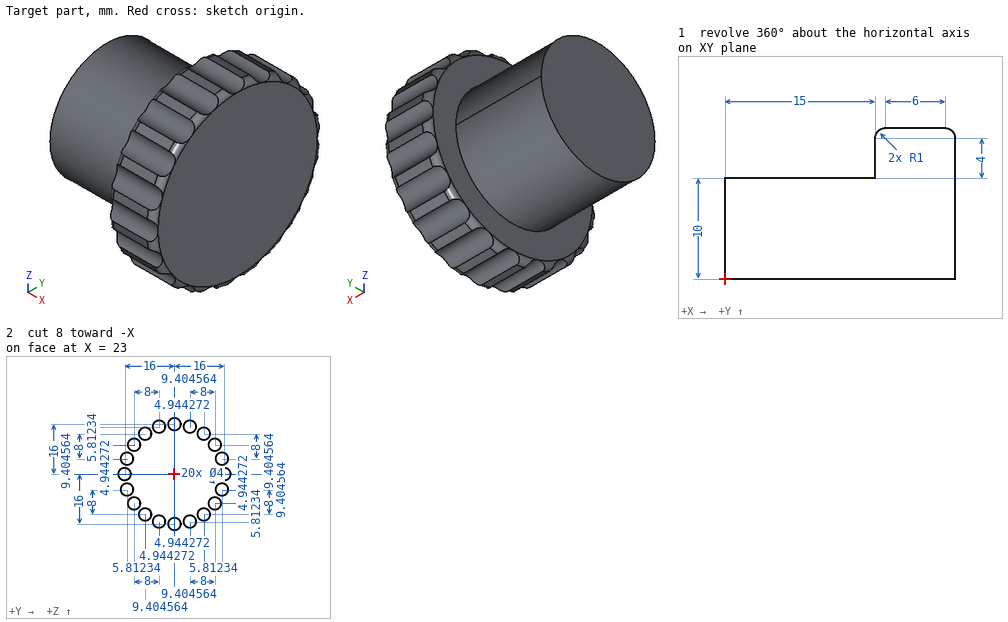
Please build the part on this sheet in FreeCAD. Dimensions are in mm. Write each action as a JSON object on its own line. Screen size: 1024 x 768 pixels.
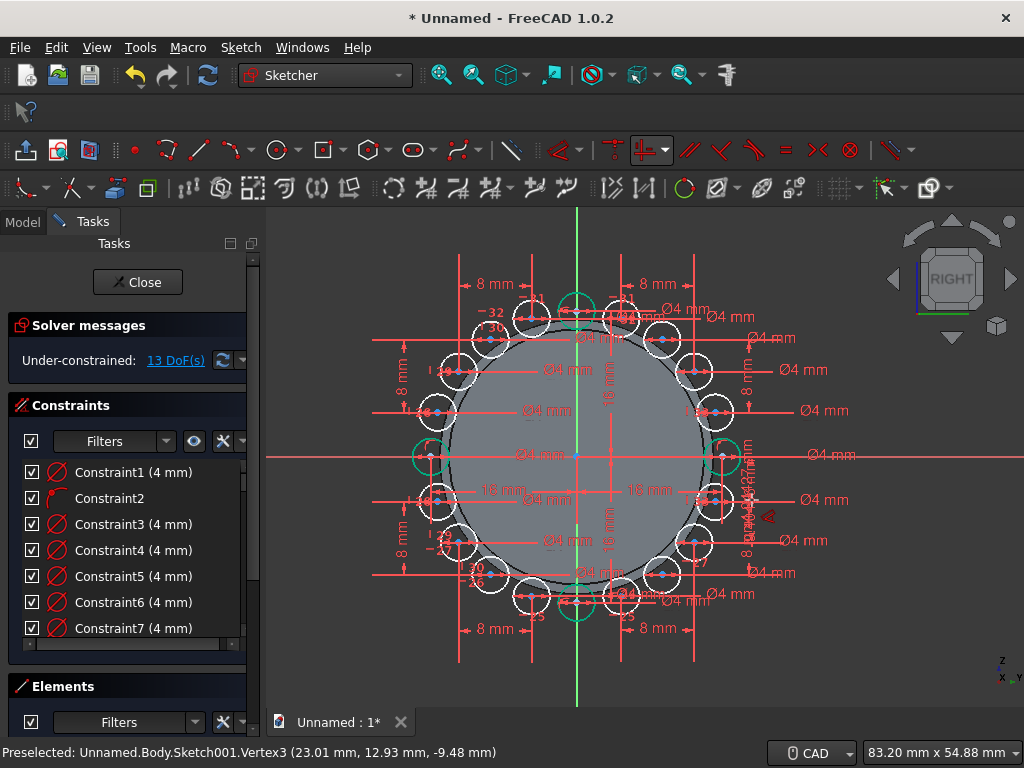
{"action": "left_click", "coordinate": [662, 575]}
{"action": "left_click", "coordinate": [619, 423]}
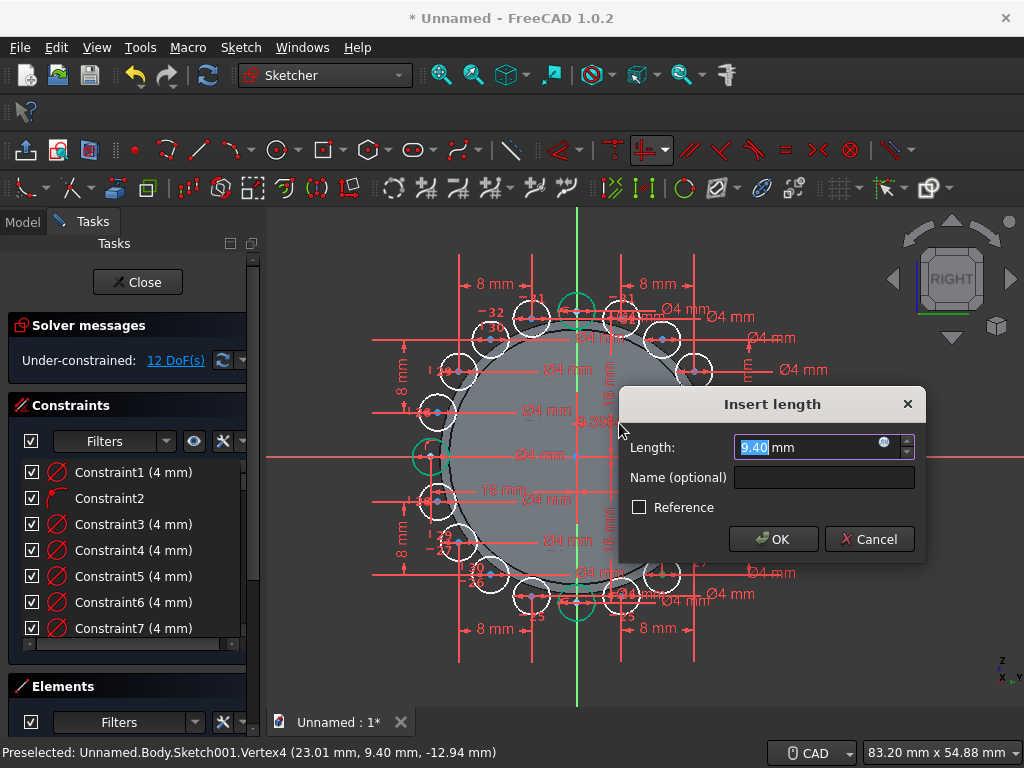
{"action": "type", "text": "9.404564"}
{"action": "key", "text": "Return"}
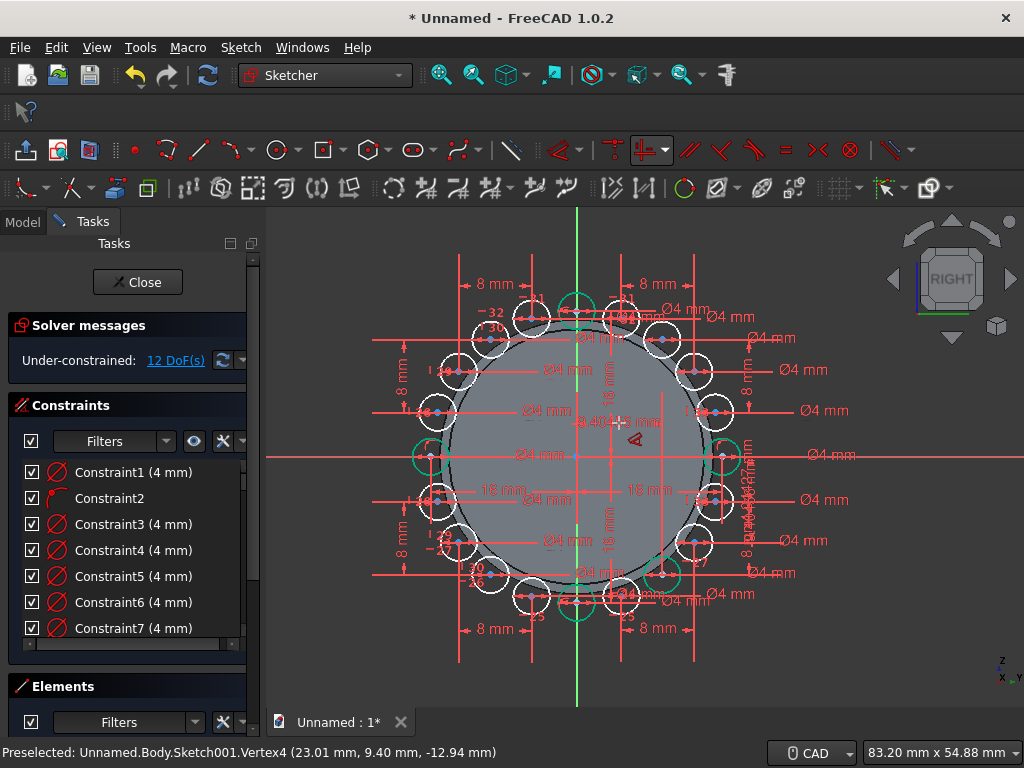
{"action": "left_click", "coordinate": [621, 596]}
{"action": "left_click", "coordinate": [599, 654]}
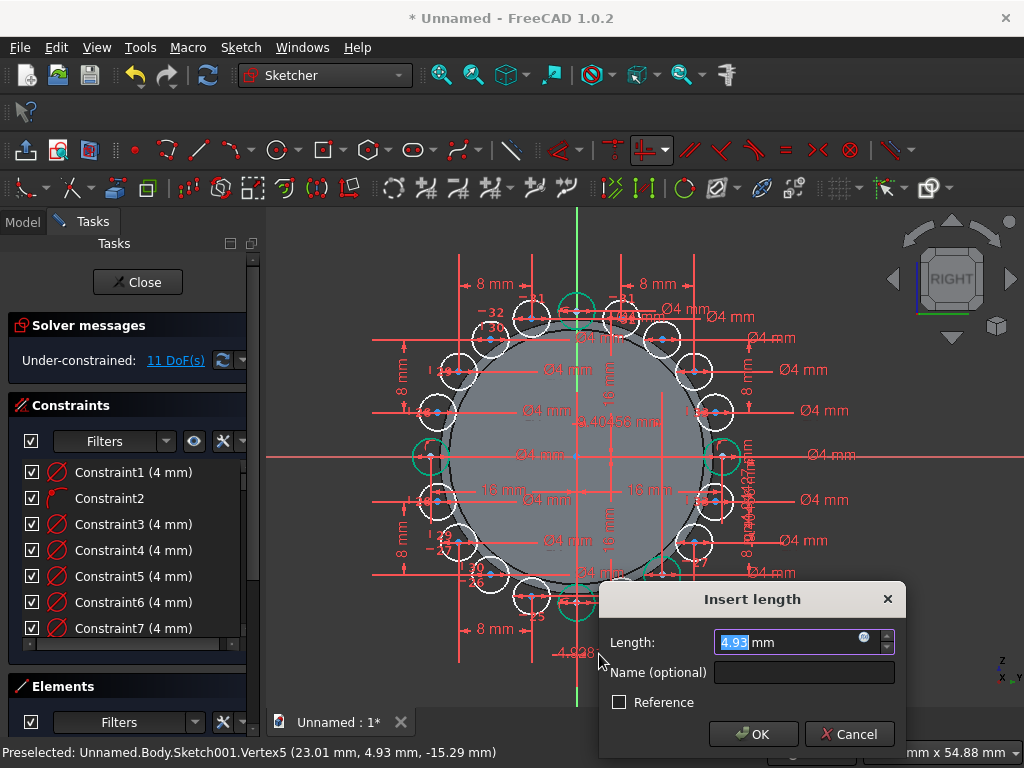
{"action": "type", "text": "4.944272"}
{"action": "key", "text": "Return"}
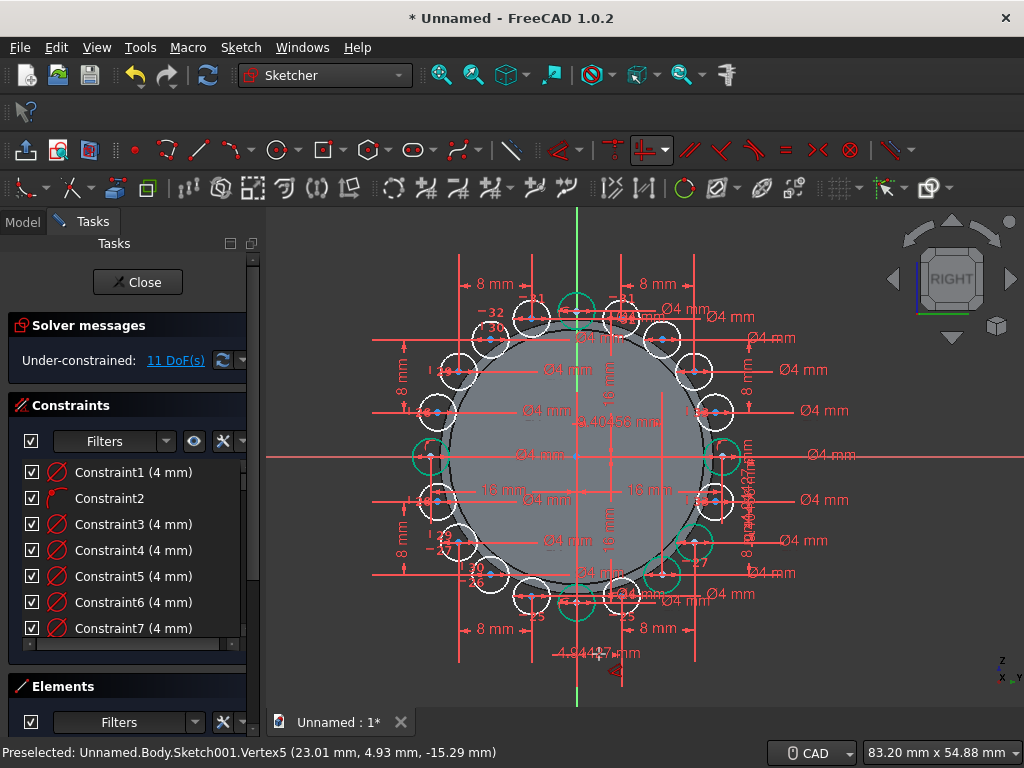
{"action": "left_click", "coordinate": [532, 596]}
{"action": "left_click", "coordinate": [544, 423]}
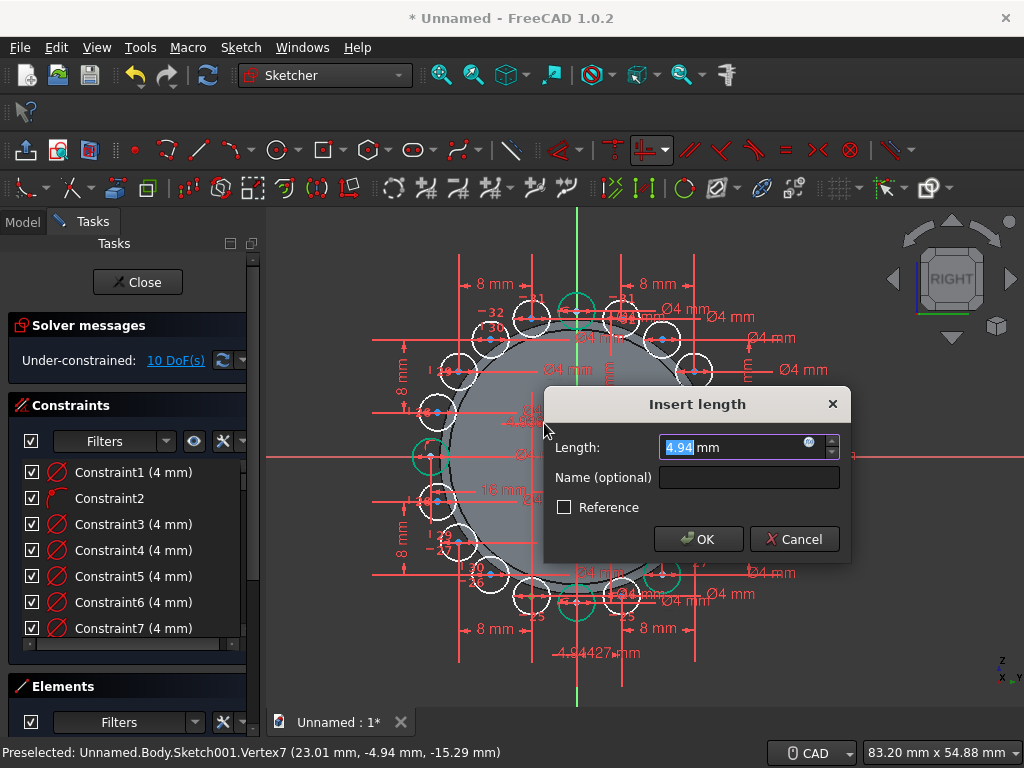
{"action": "type", "text": "4.944272"}
{"action": "key", "text": "Return"}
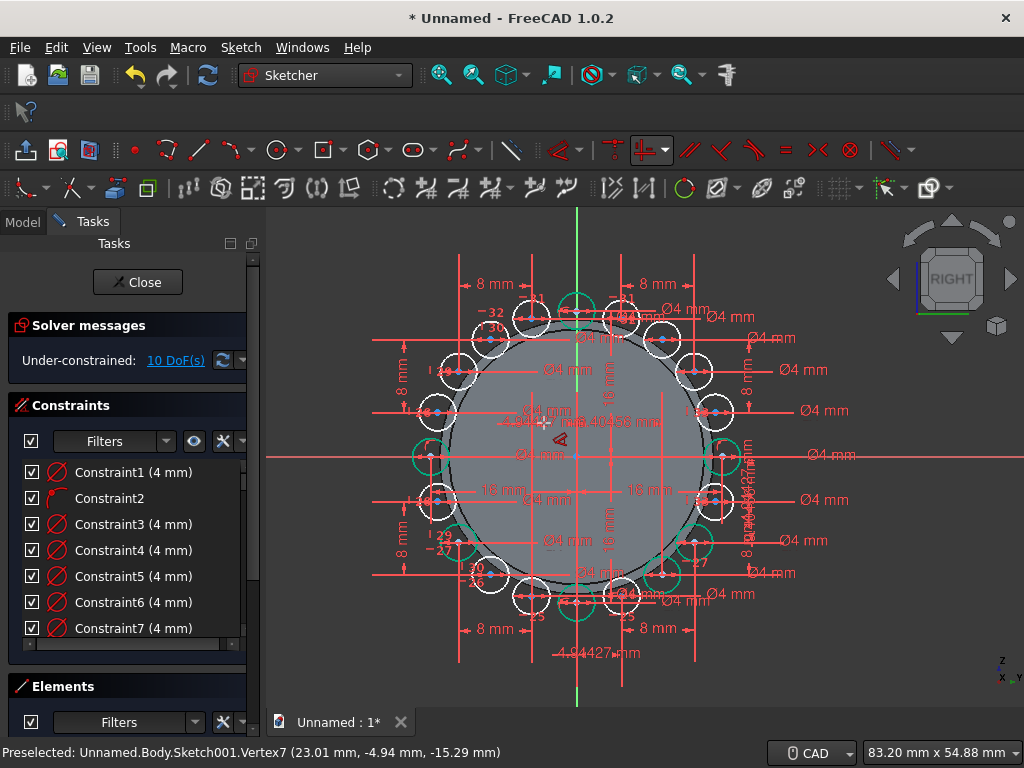
{"action": "left_click", "coordinate": [491, 575]}
{"action": "left_click", "coordinate": [534, 399]}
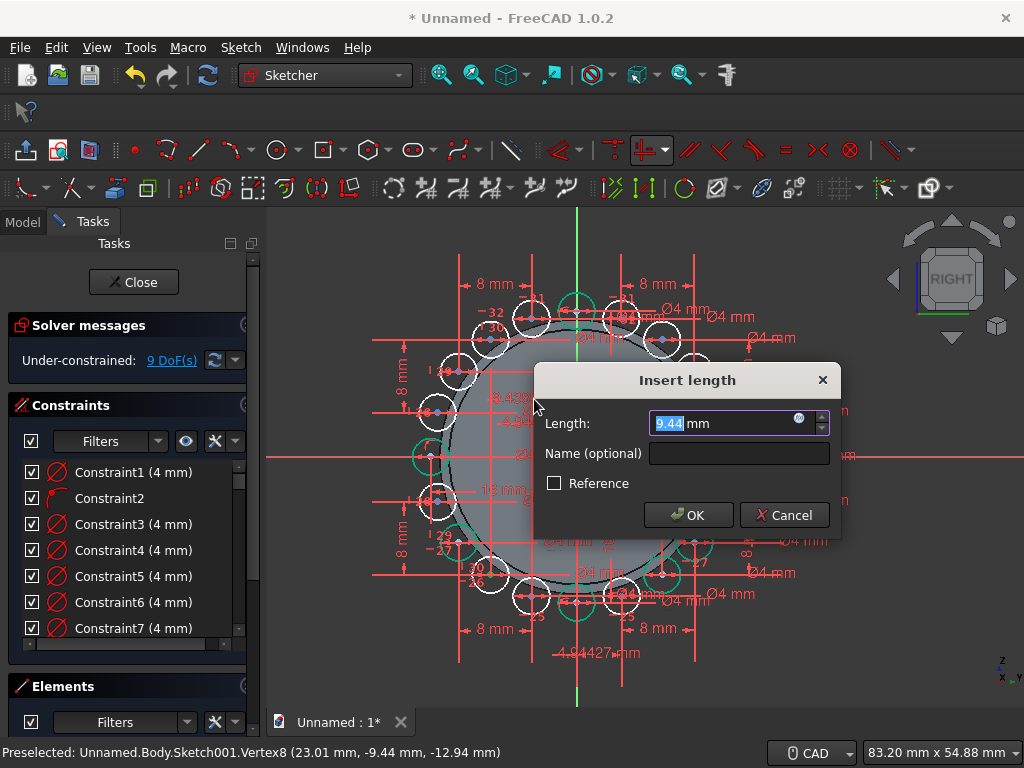
{"action": "type", "text": "9.404564"}
{"action": "key", "text": "Return"}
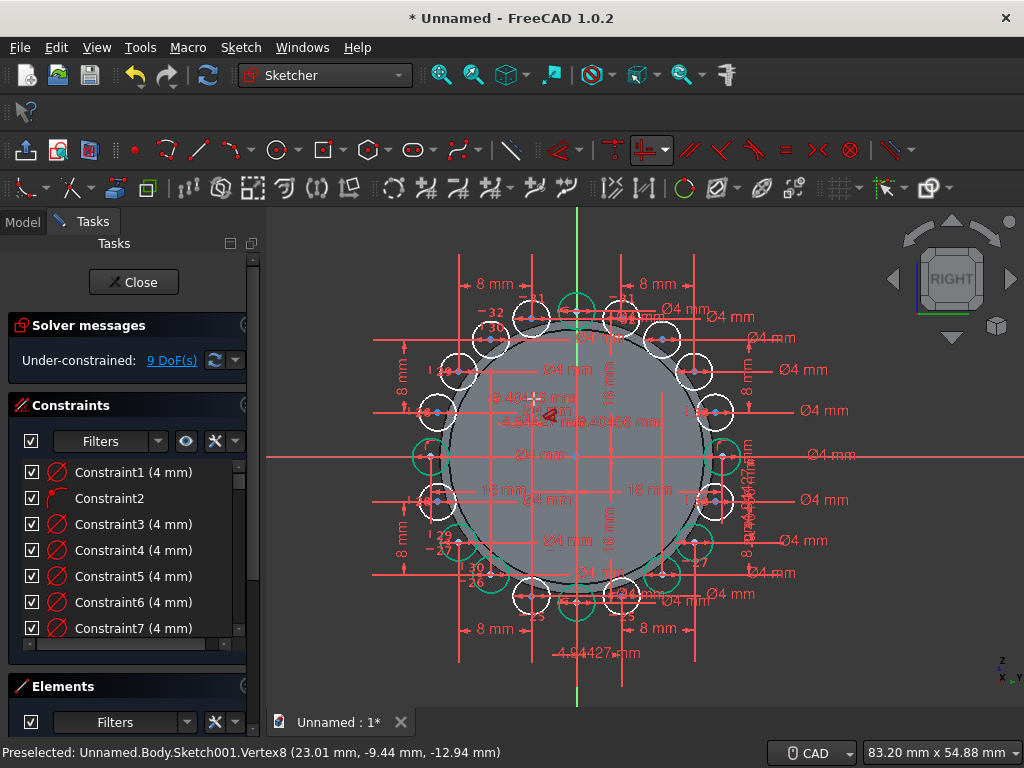
{"action": "left_click", "coordinate": [438, 413]}
{"action": "left_click", "coordinate": [404, 435]}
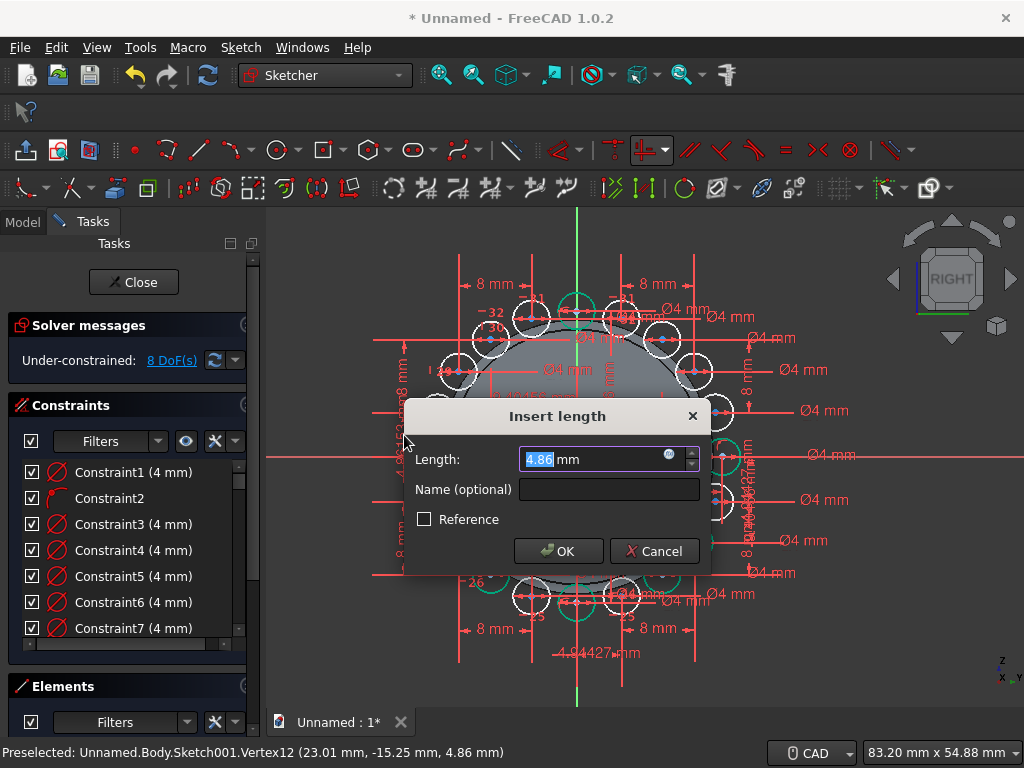
{"action": "type", "text": "4.944272"}
{"action": "key", "text": "Return"}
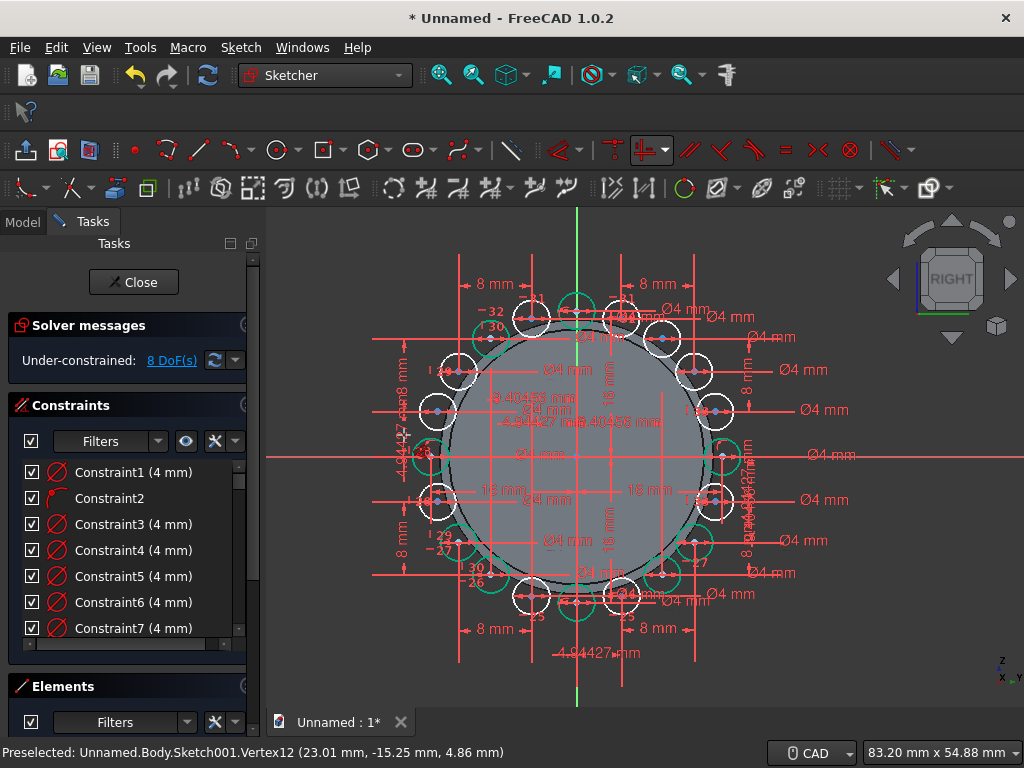
{"action": "left_click", "coordinate": [459, 372]}
{"action": "left_click", "coordinate": [401, 414]}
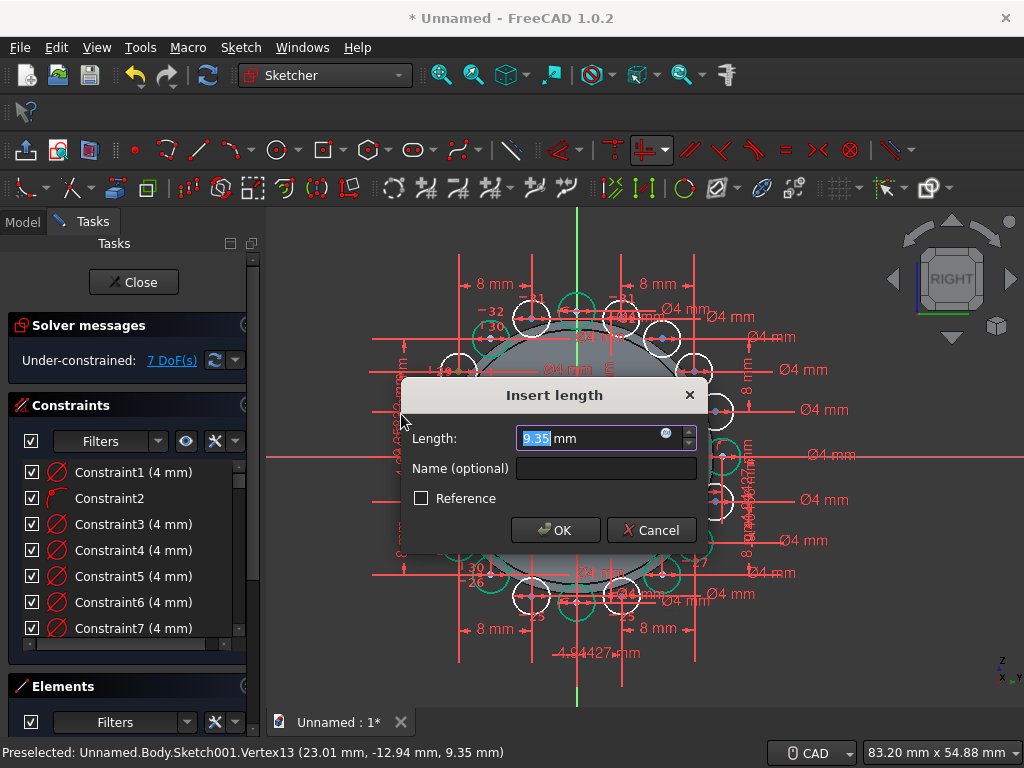
{"action": "type", "text": "9.404564"}
{"action": "key", "text": "Return"}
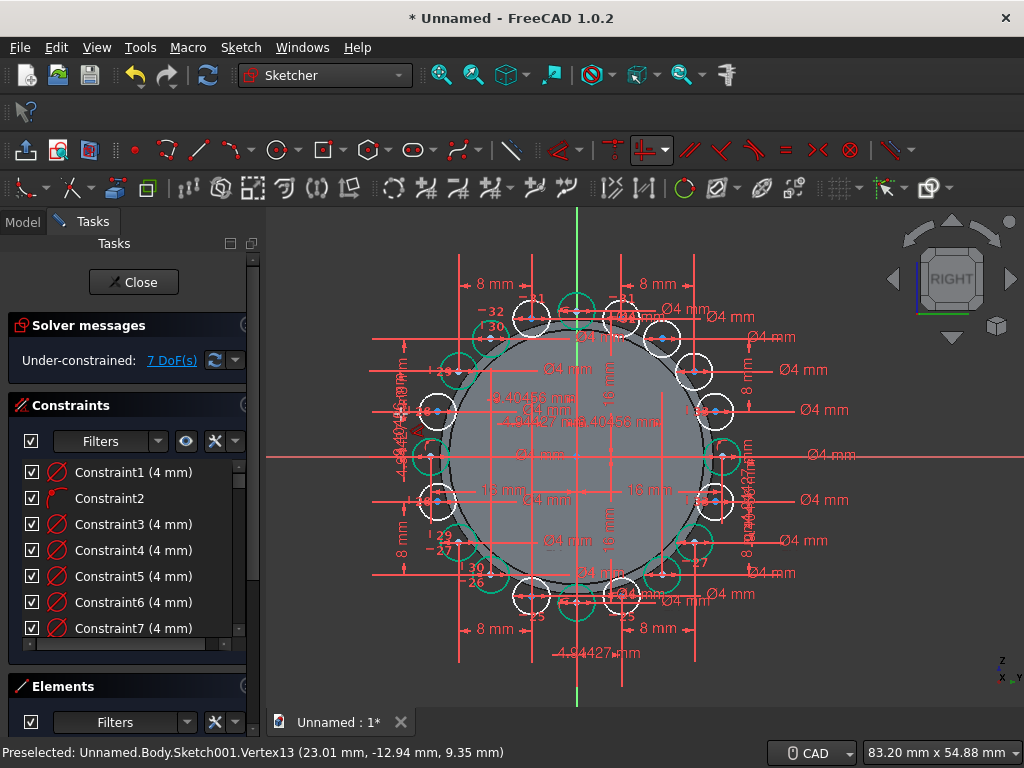
{"action": "left_click", "coordinate": [621, 319]}
{"action": "left_click", "coordinate": [599, 261]}